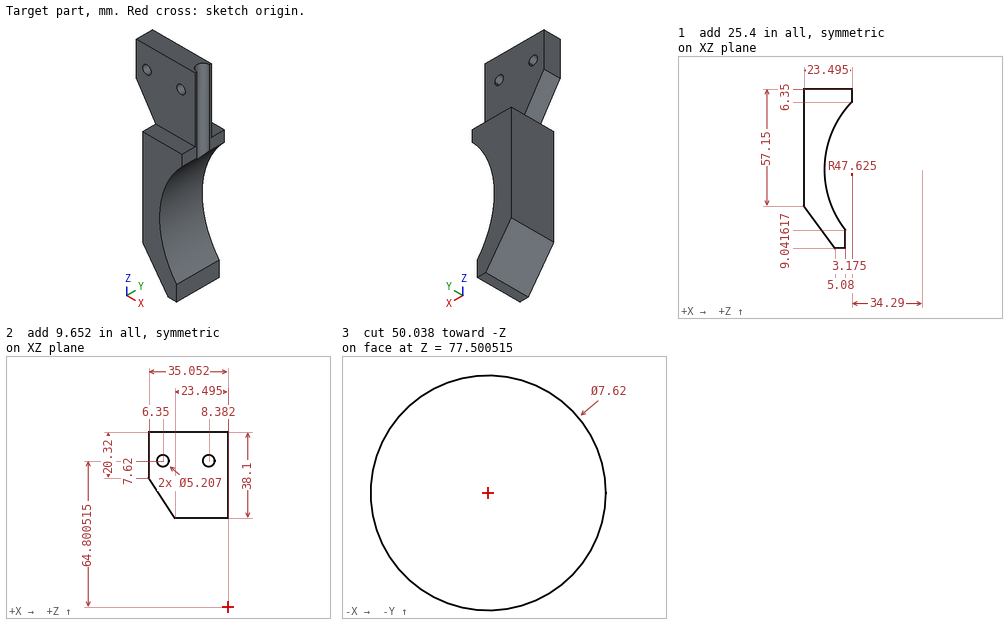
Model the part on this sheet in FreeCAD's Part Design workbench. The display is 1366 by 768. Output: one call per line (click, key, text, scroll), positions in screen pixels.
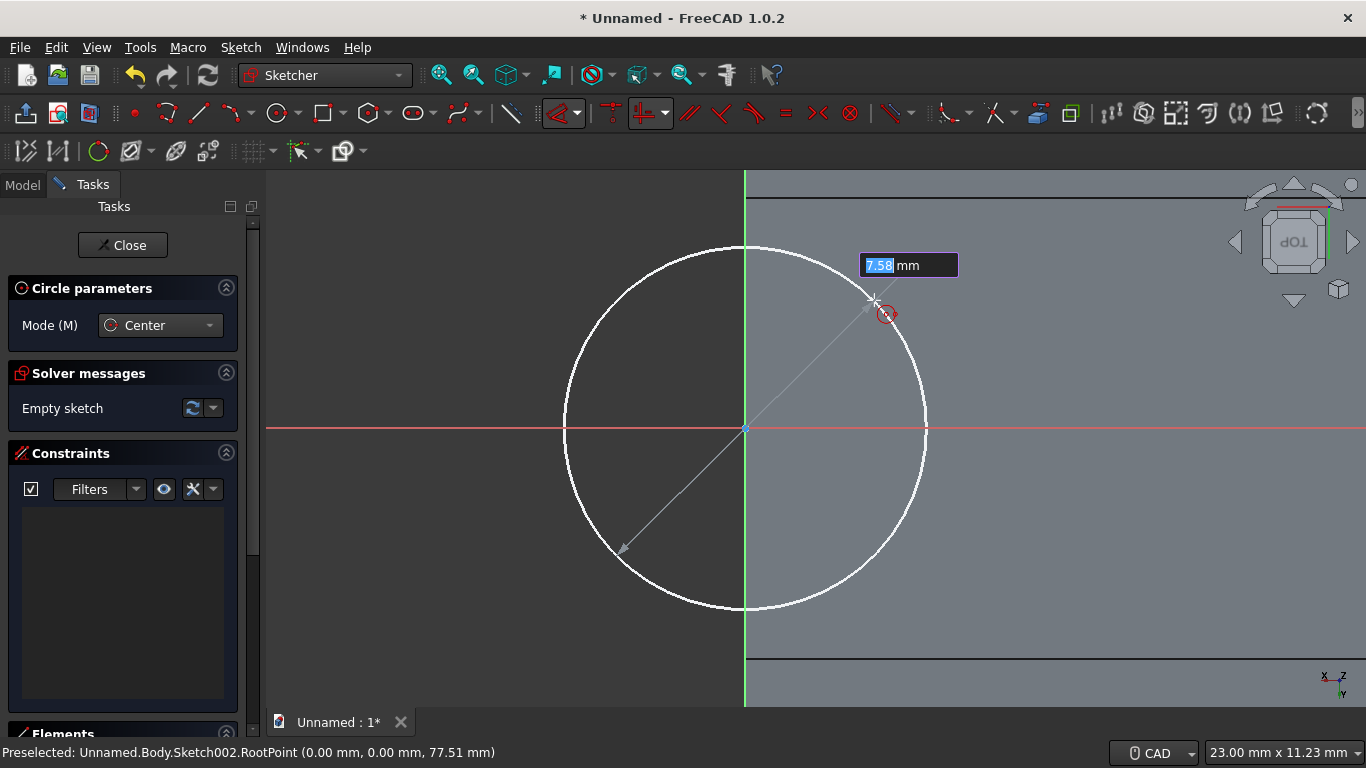
text(7.62)
key(Return)
key(Escape)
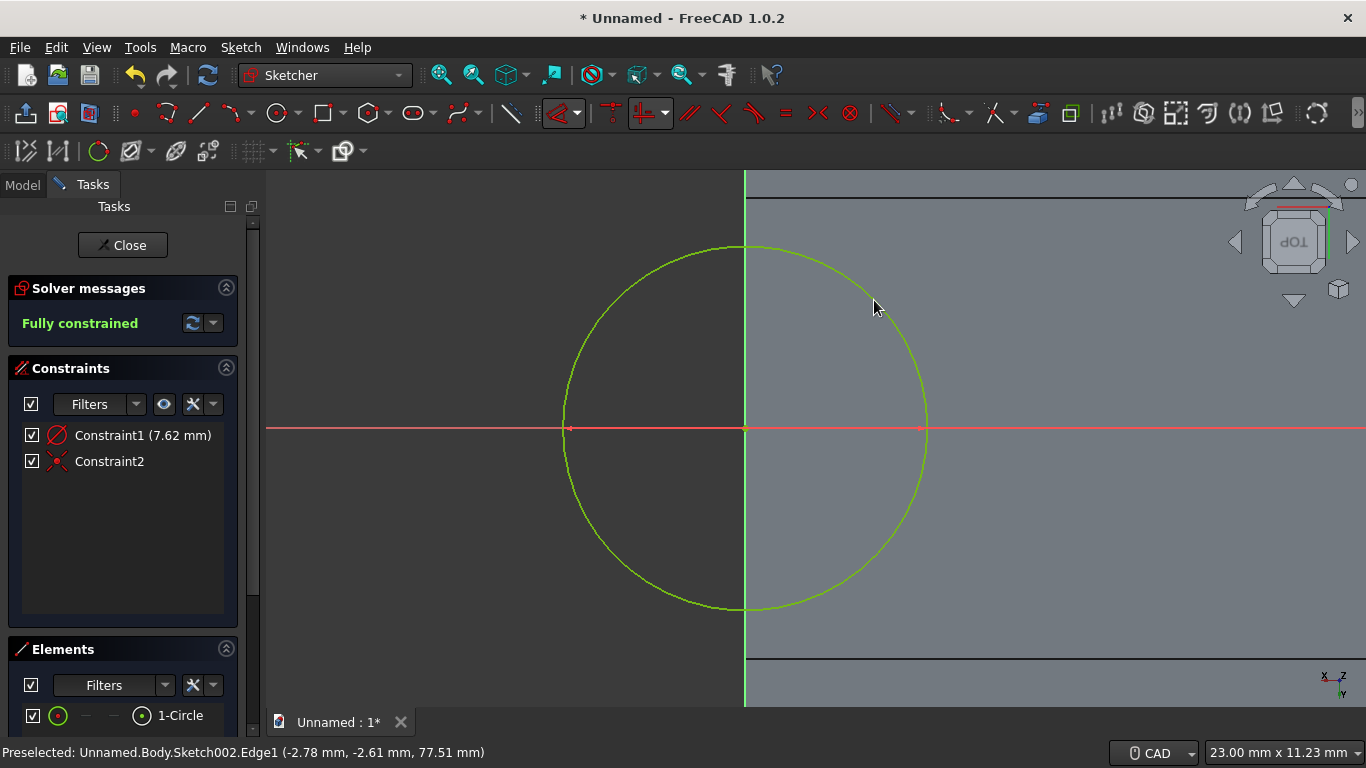
click(123, 245)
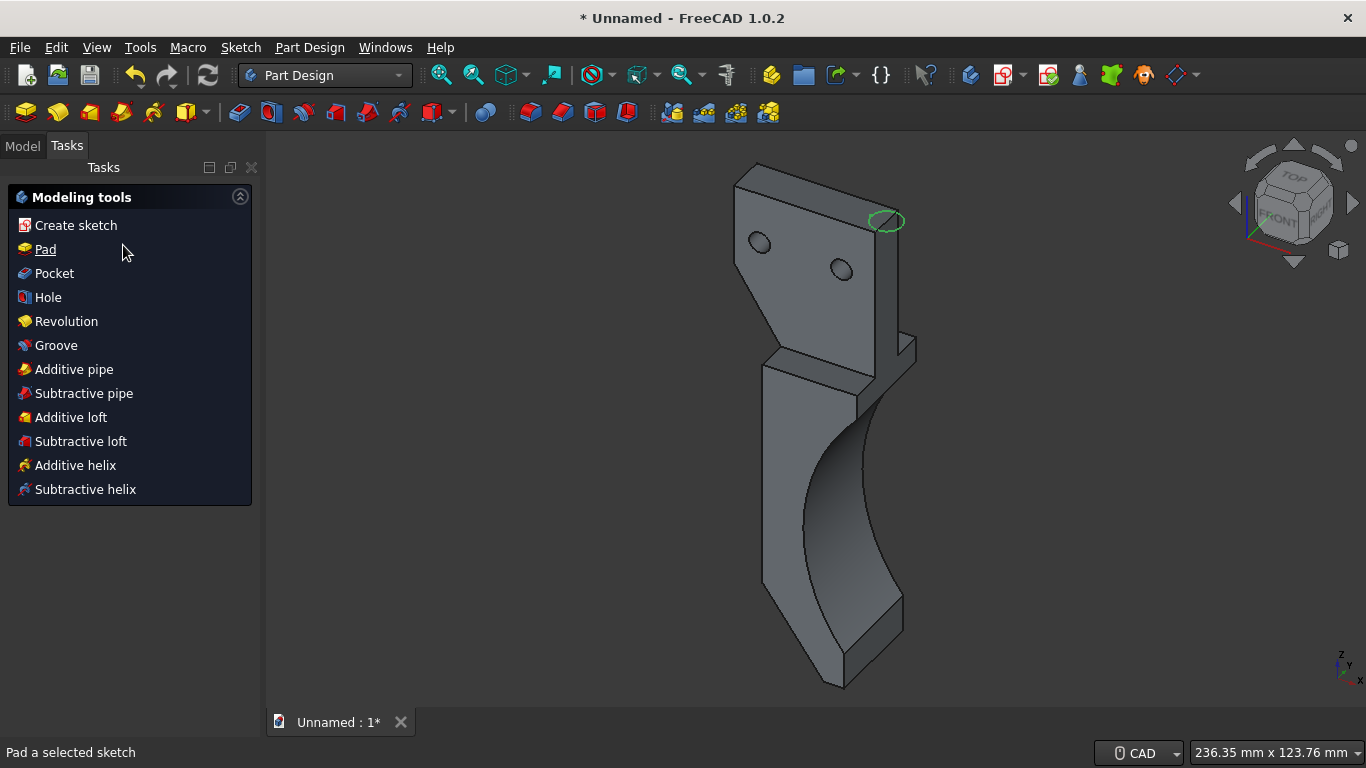
click(240, 112)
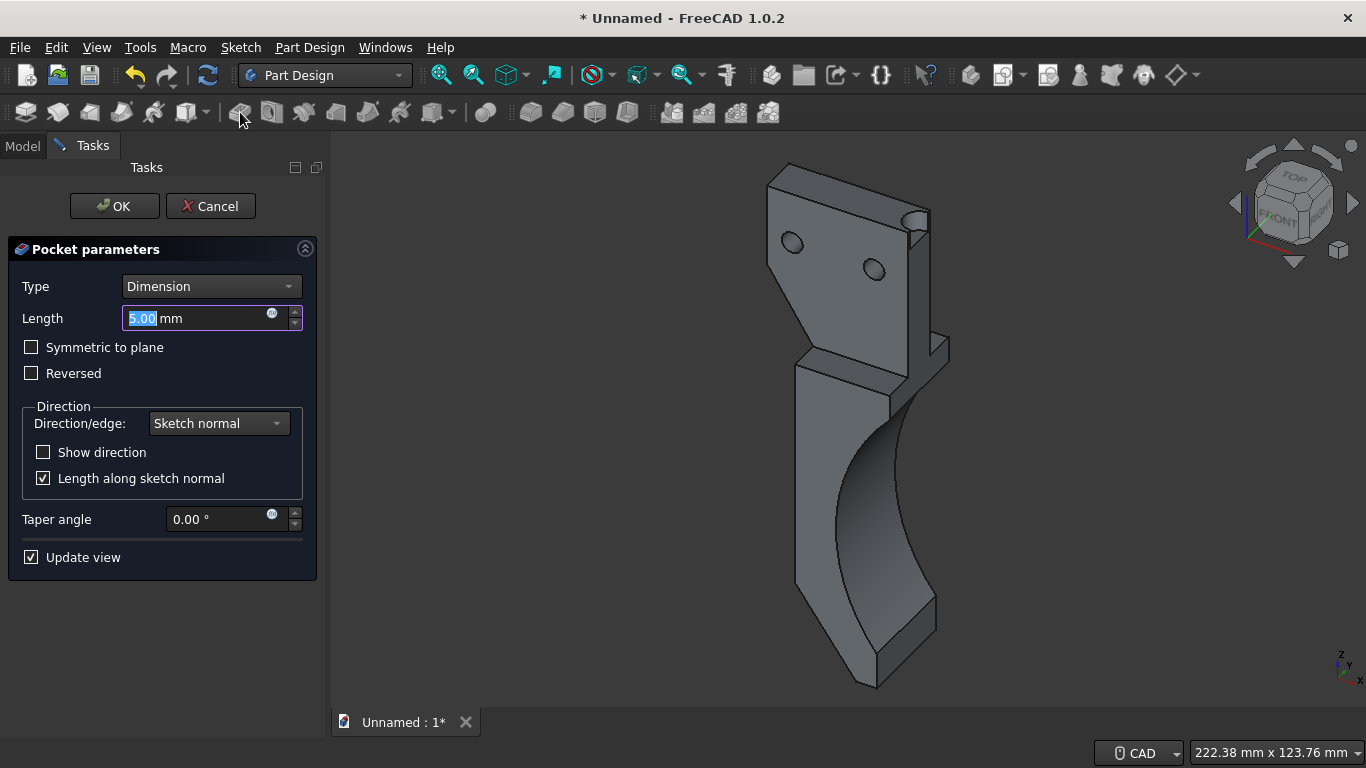
text(50.038)
key(Tab)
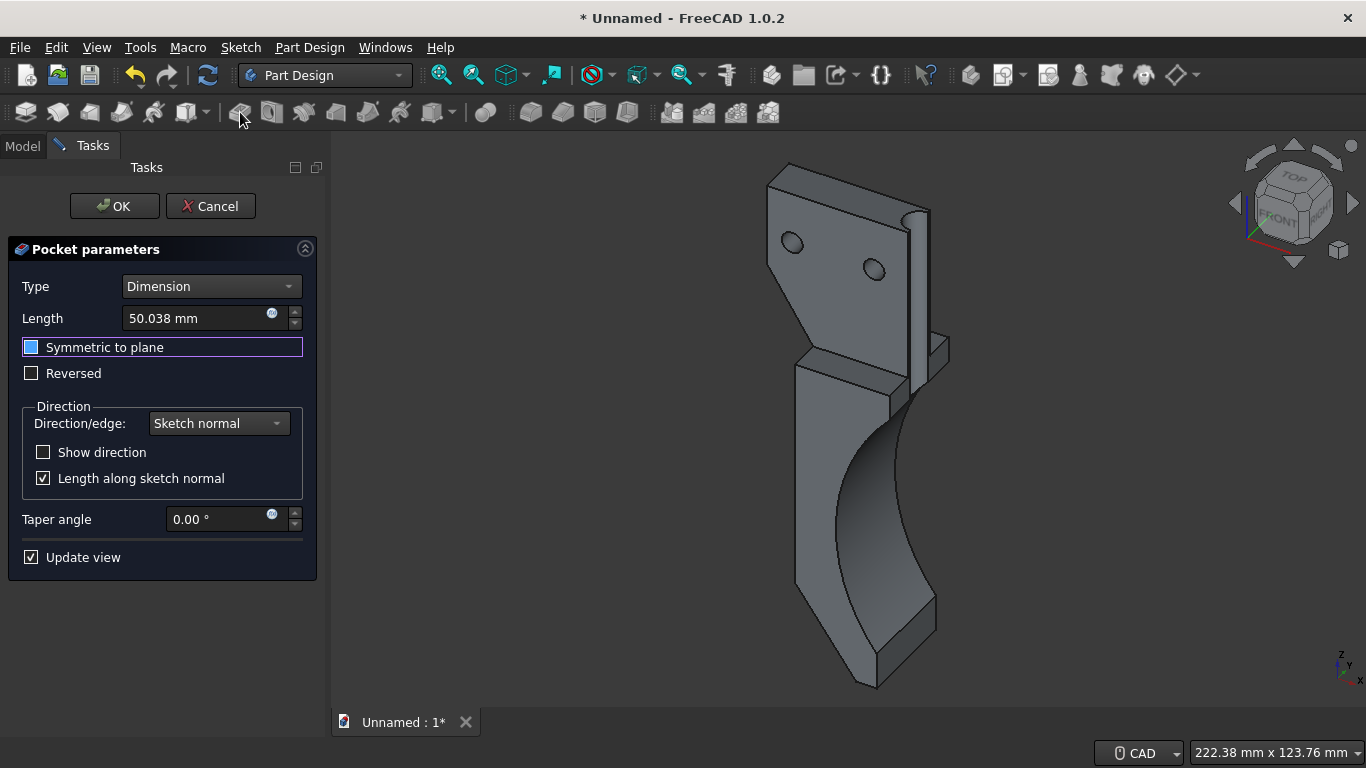
click(115, 206)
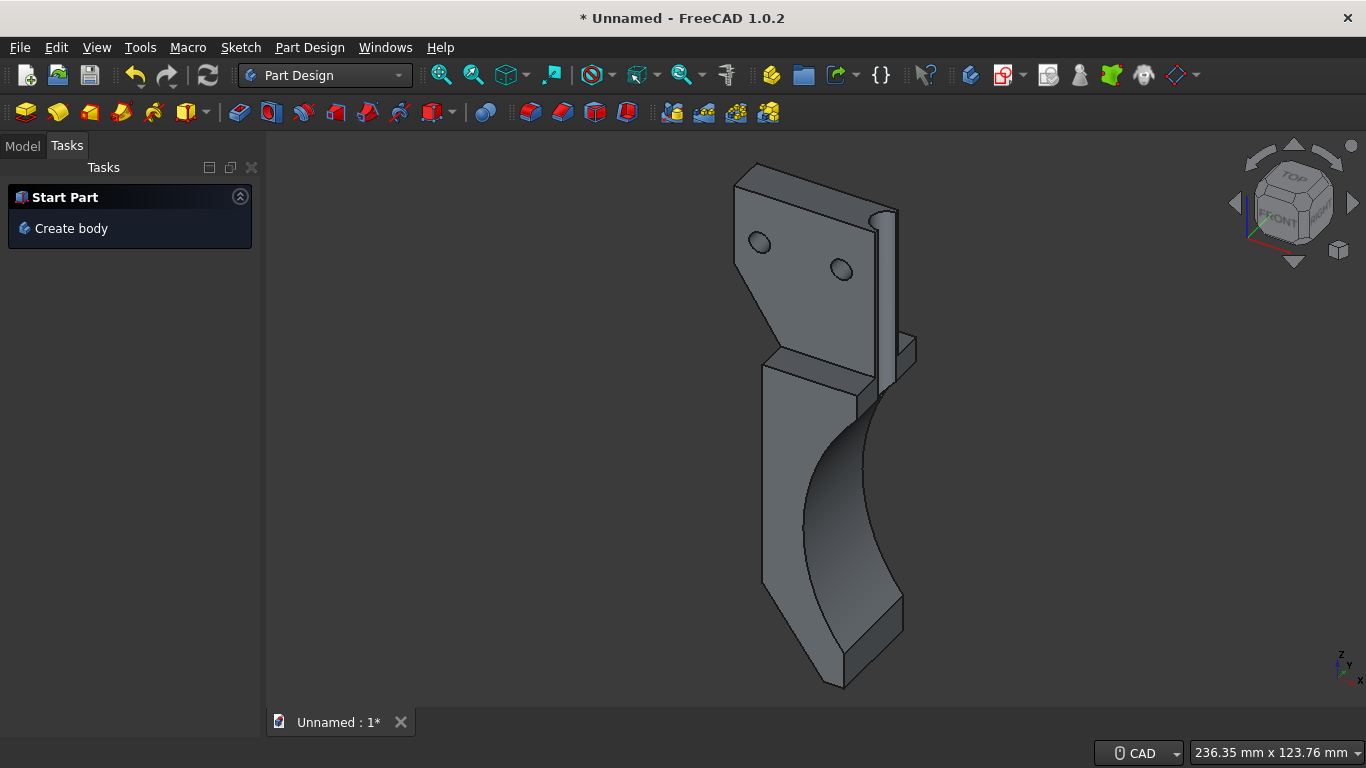
key(0)